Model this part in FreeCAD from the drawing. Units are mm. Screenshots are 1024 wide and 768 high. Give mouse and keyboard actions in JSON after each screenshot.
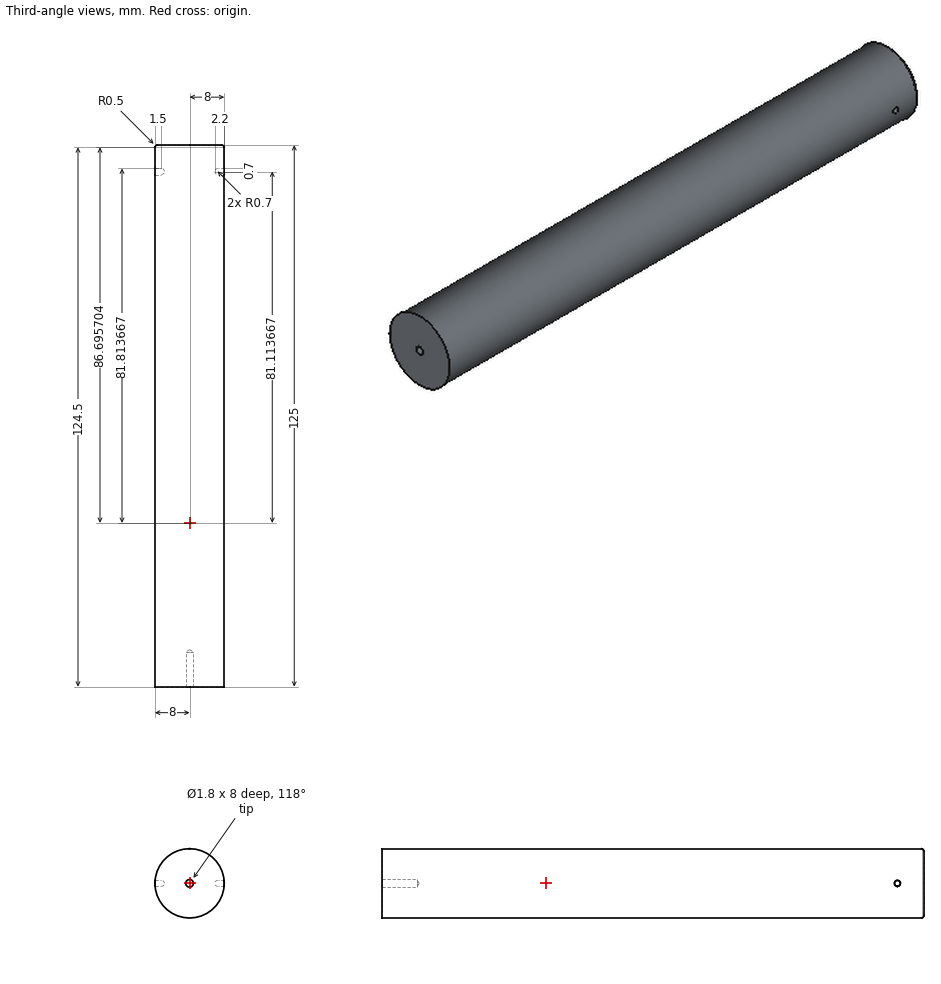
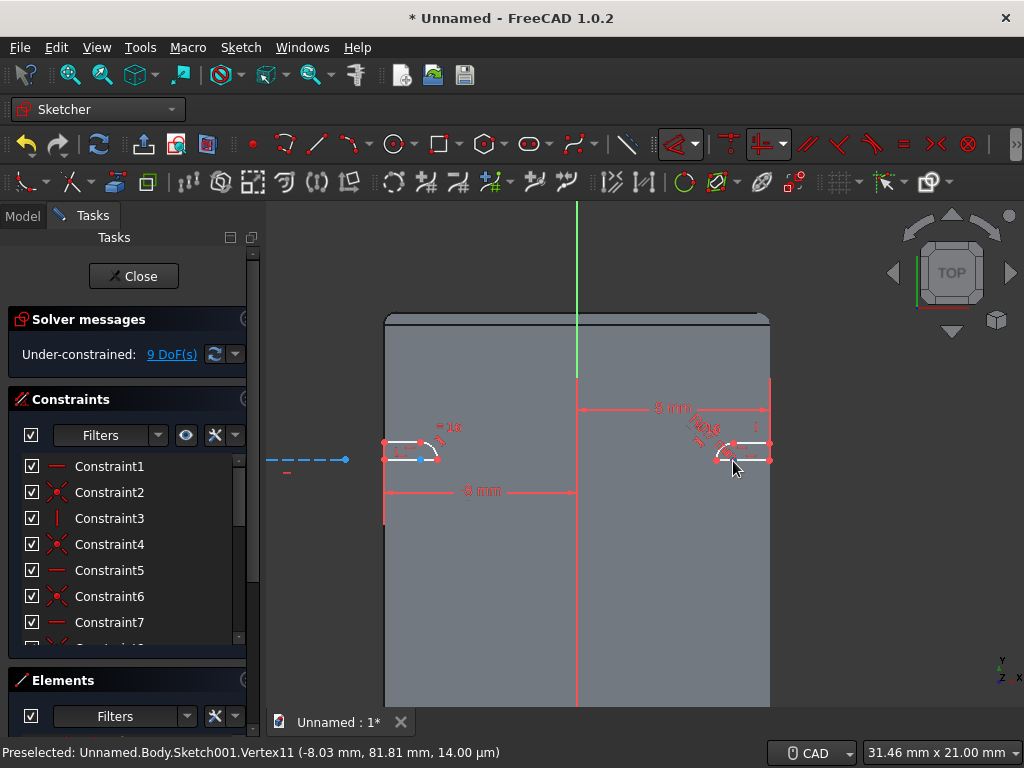
{"action": "left_click", "coordinate": [738, 460]}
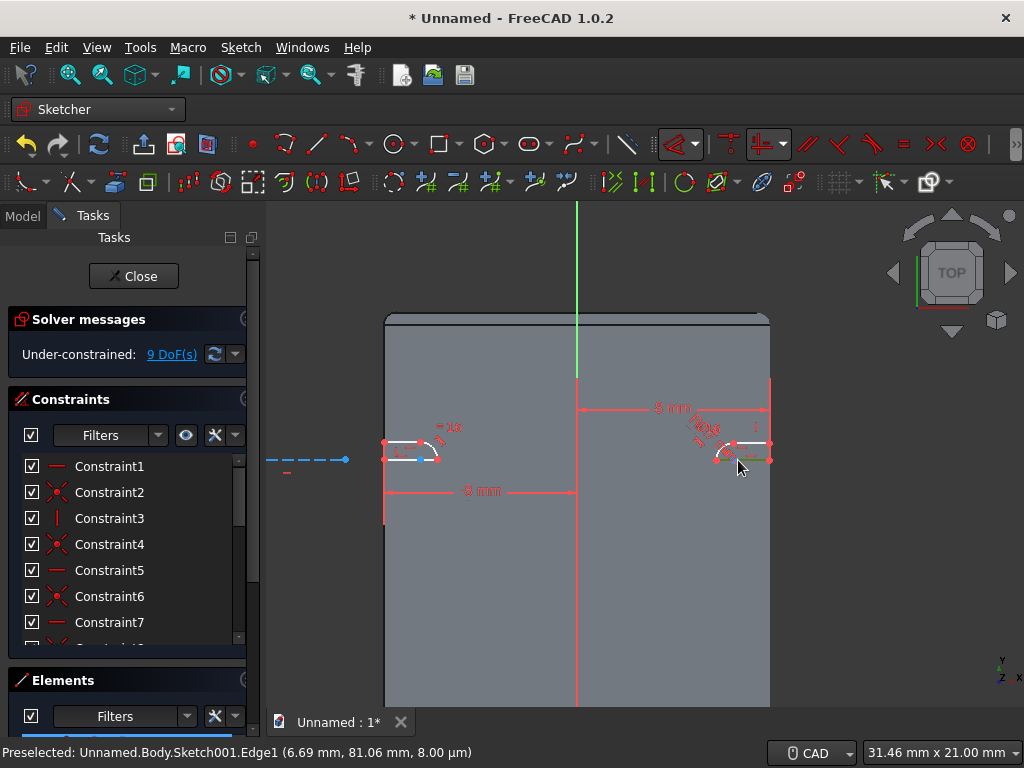
{"action": "left_click", "coordinate": [698, 144]}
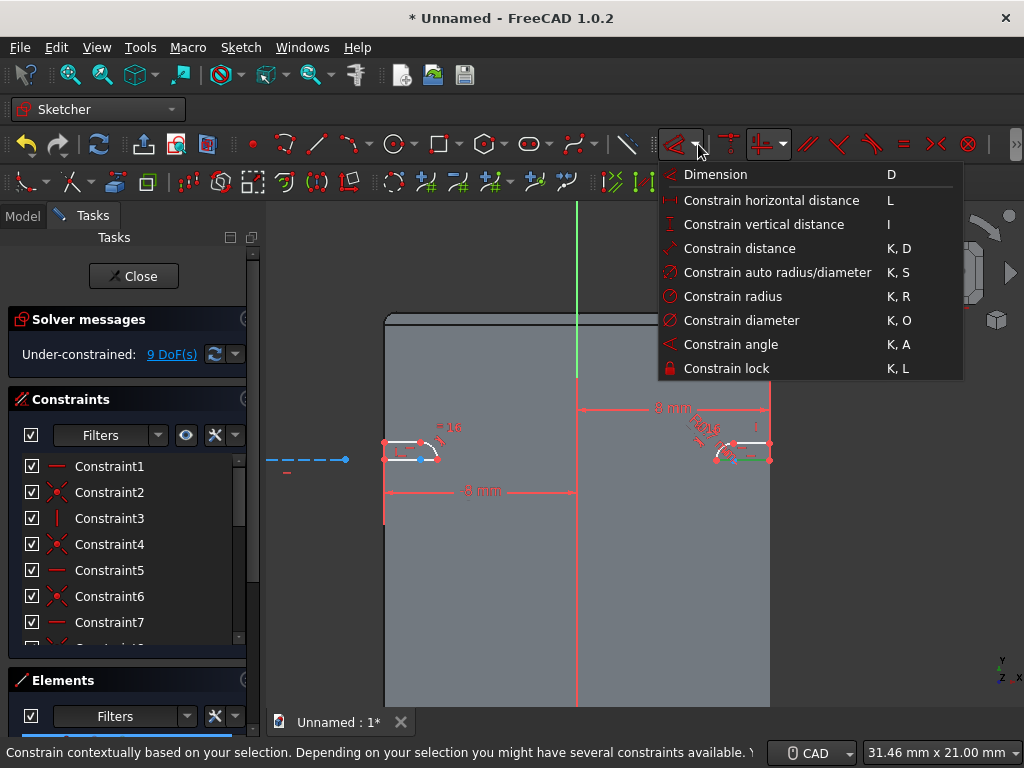
{"action": "left_click", "coordinate": [811, 200]}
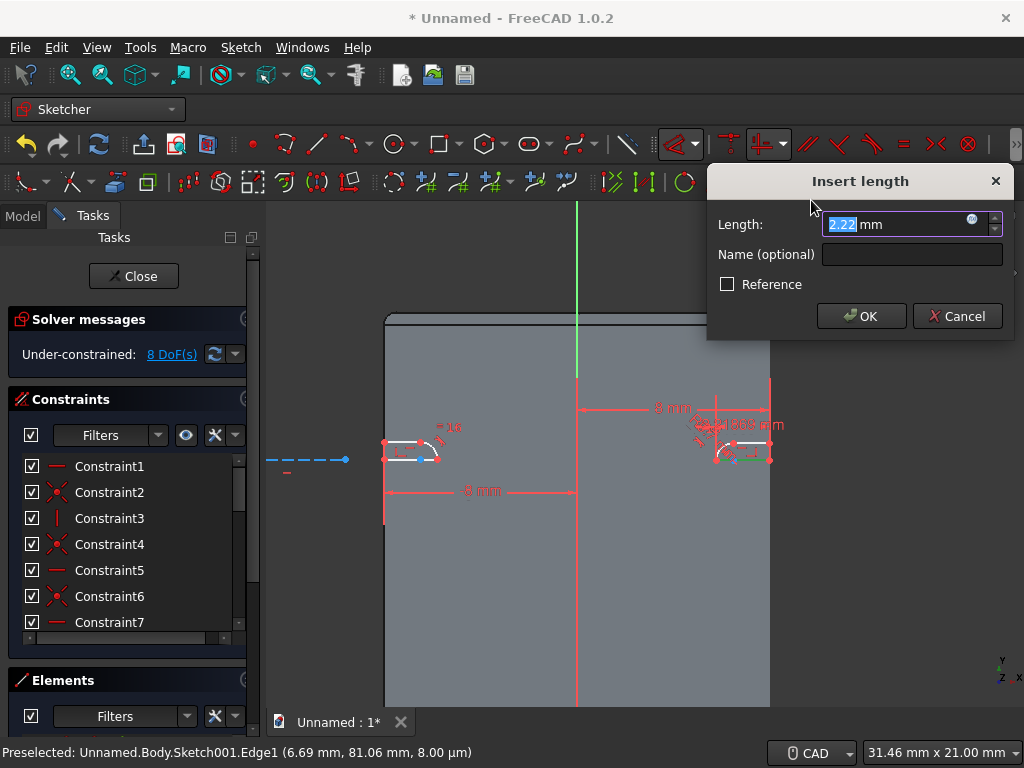
{"action": "type", "text": "2.2"}
{"action": "key", "text": "Return"}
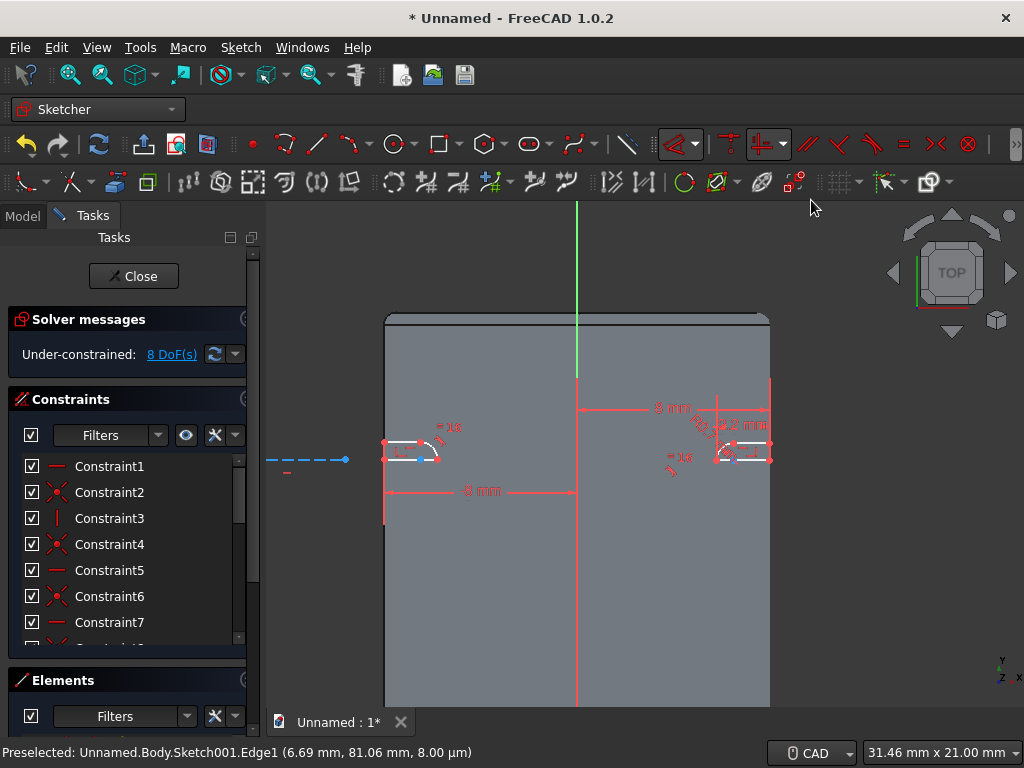
{"action": "scroll", "coordinate": [770, 452], "scroll_direction": "up", "scroll_amount": 5}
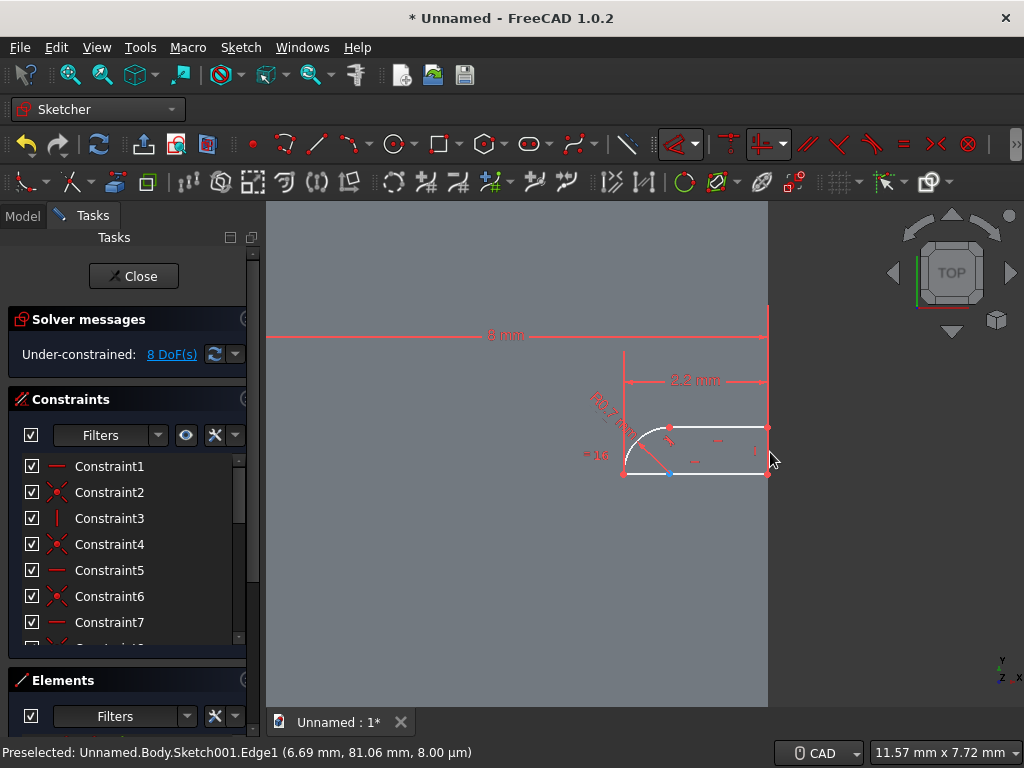
{"action": "left_click", "coordinate": [768, 451]}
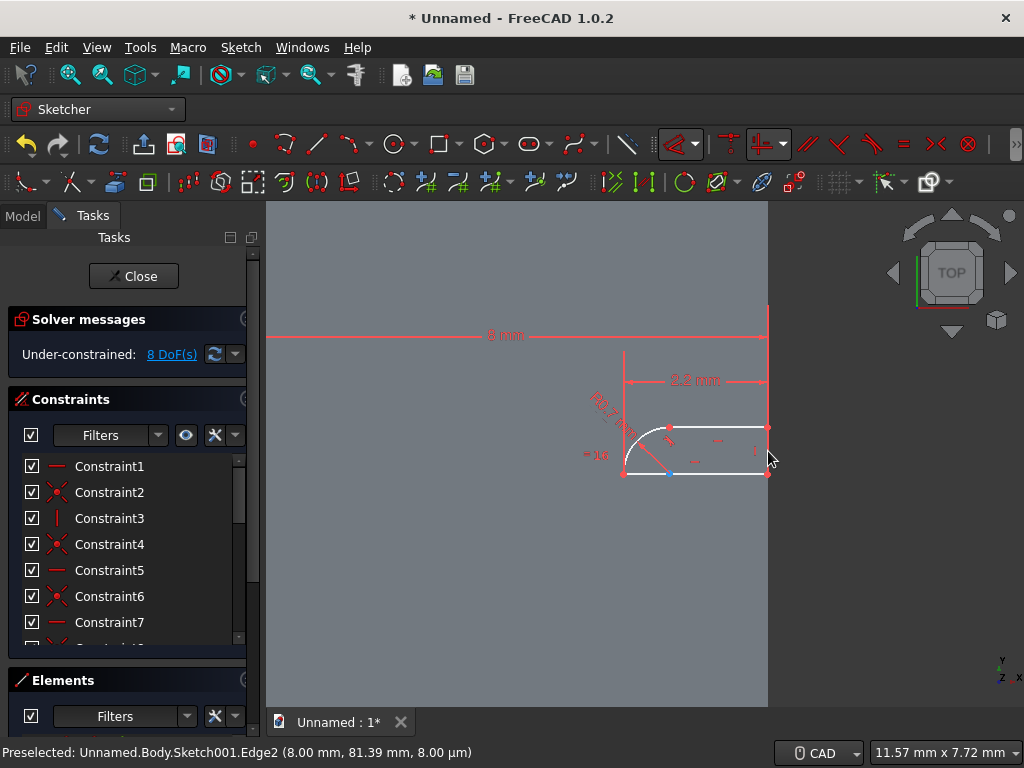
{"action": "left_click", "coordinate": [698, 144]}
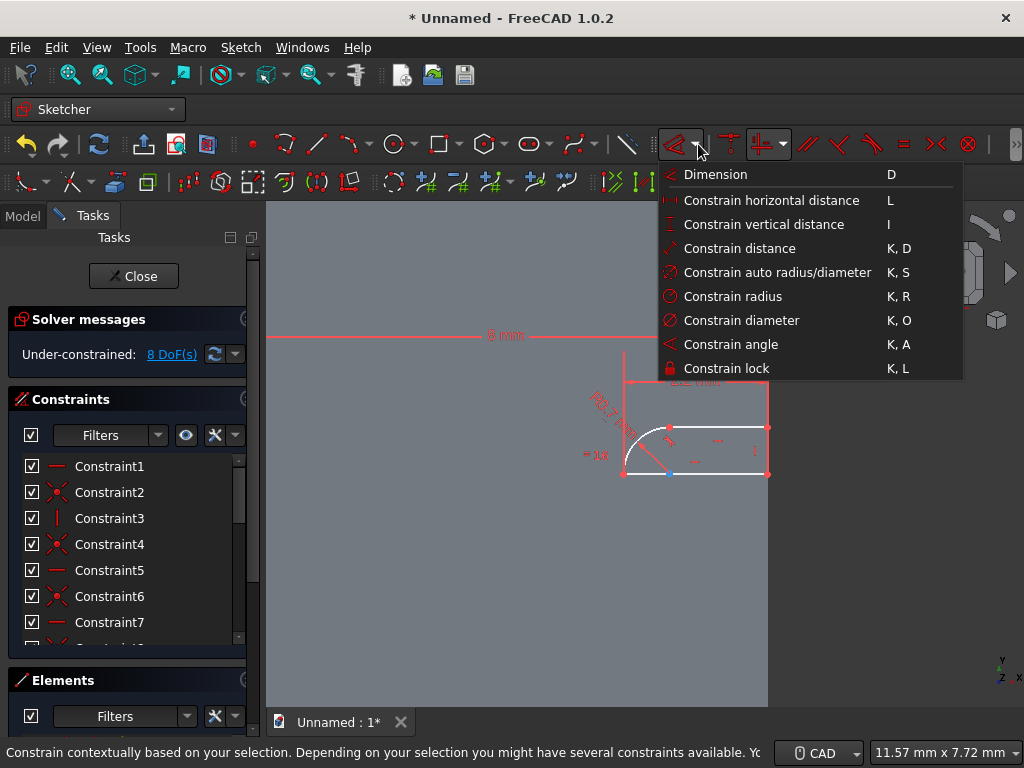
{"action": "left_click", "coordinate": [811, 224]}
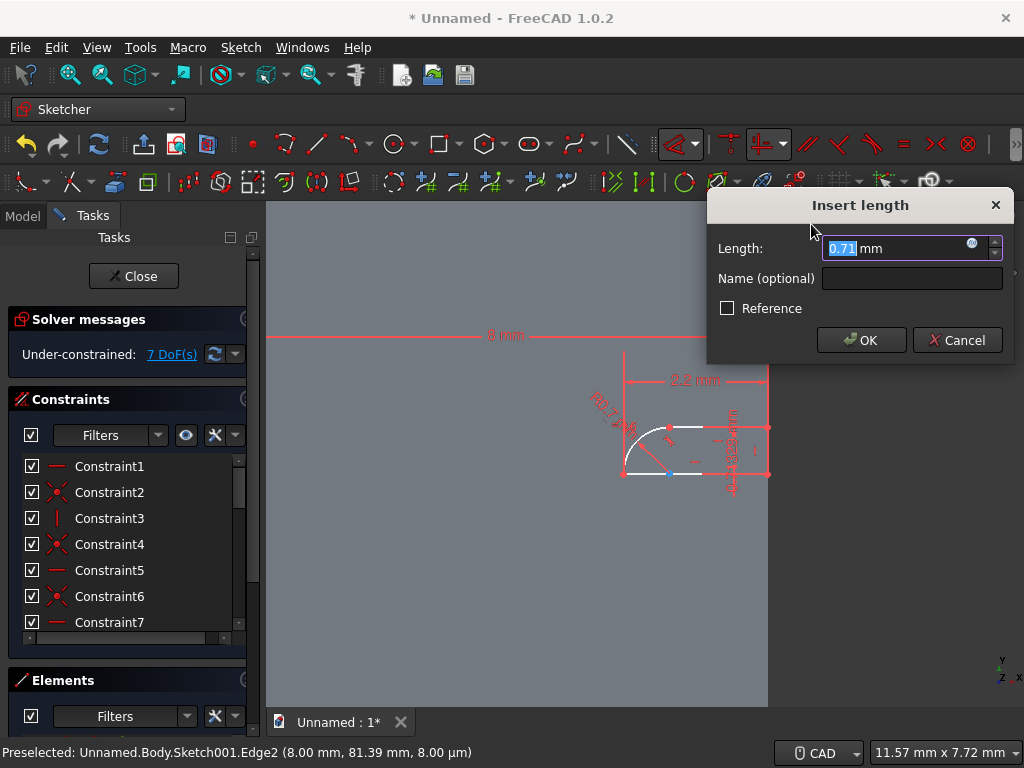
{"action": "type", "text": "0.7"}
{"action": "key", "text": "Return"}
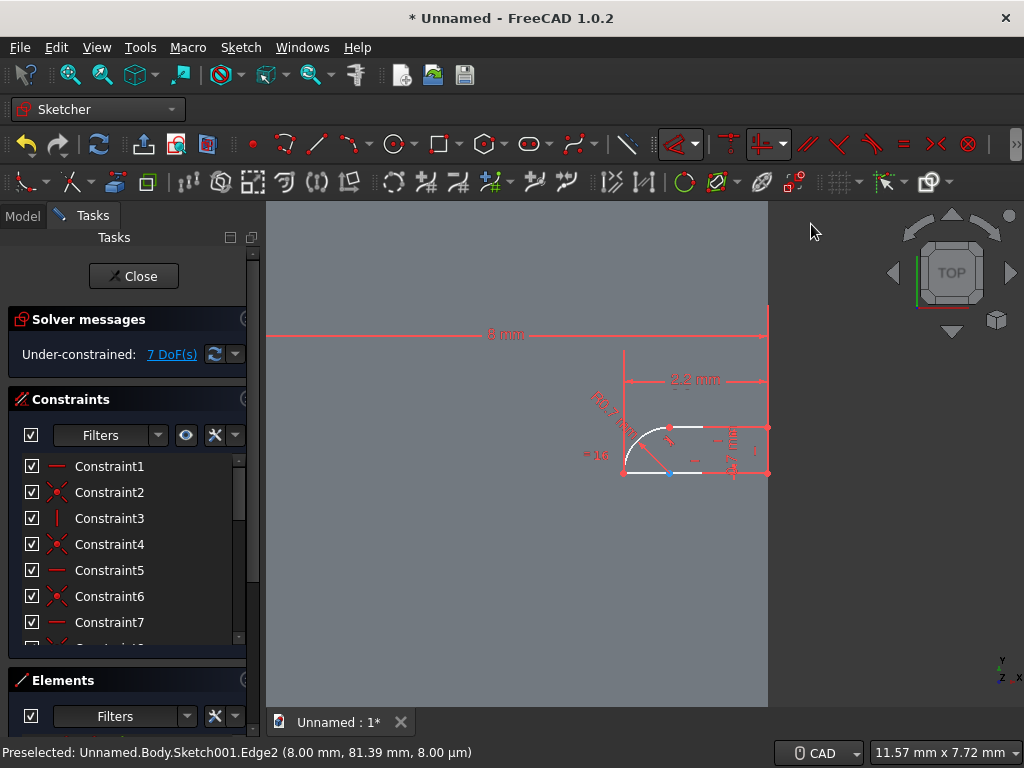
{"action": "scroll", "coordinate": [754, 456], "scroll_direction": "down", "scroll_amount": 7}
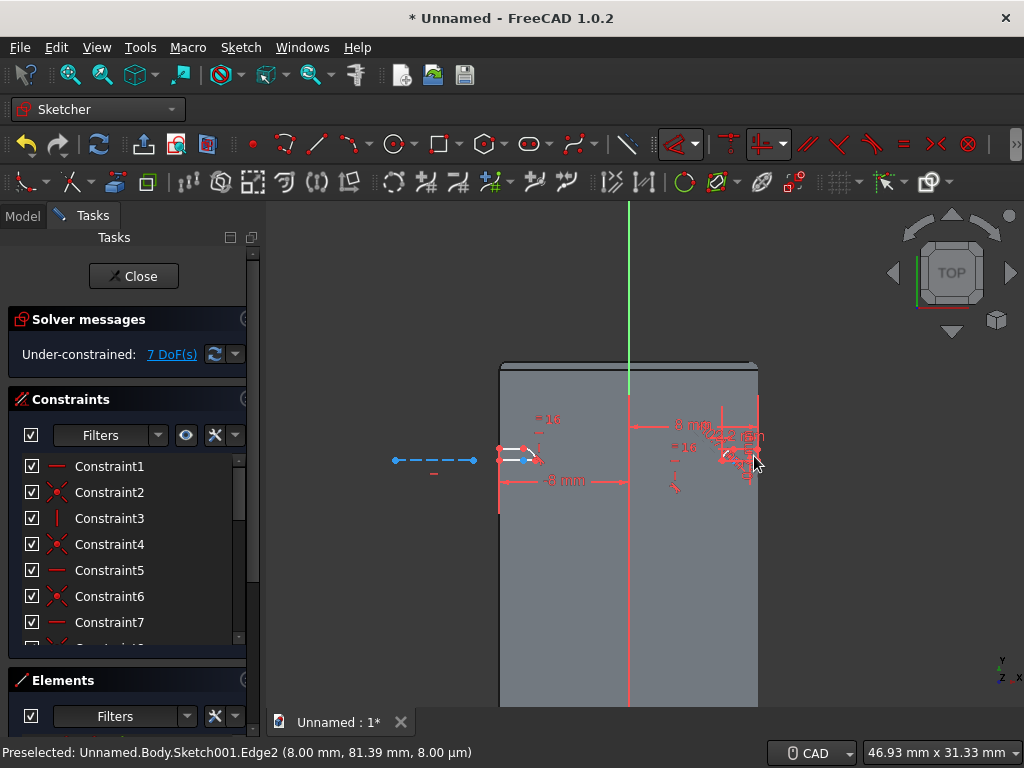
{"action": "scroll", "coordinate": [517, 449], "scroll_direction": "up", "scroll_amount": 4}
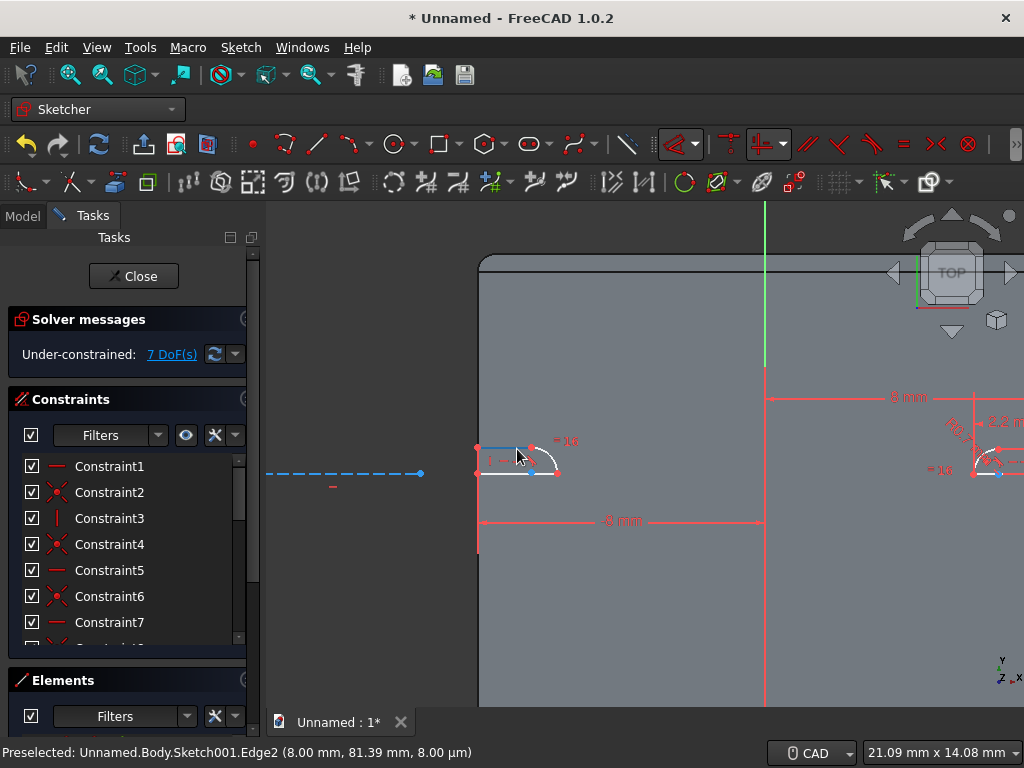
{"action": "left_click", "coordinate": [516, 448]}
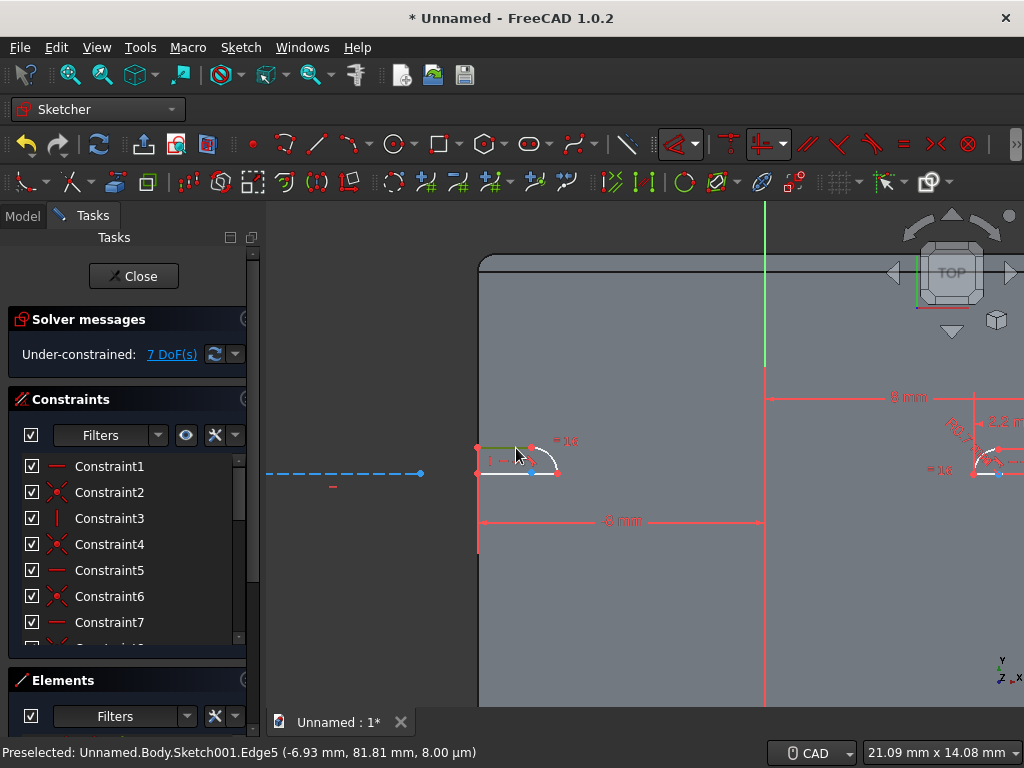
{"action": "key", "text": "l"}